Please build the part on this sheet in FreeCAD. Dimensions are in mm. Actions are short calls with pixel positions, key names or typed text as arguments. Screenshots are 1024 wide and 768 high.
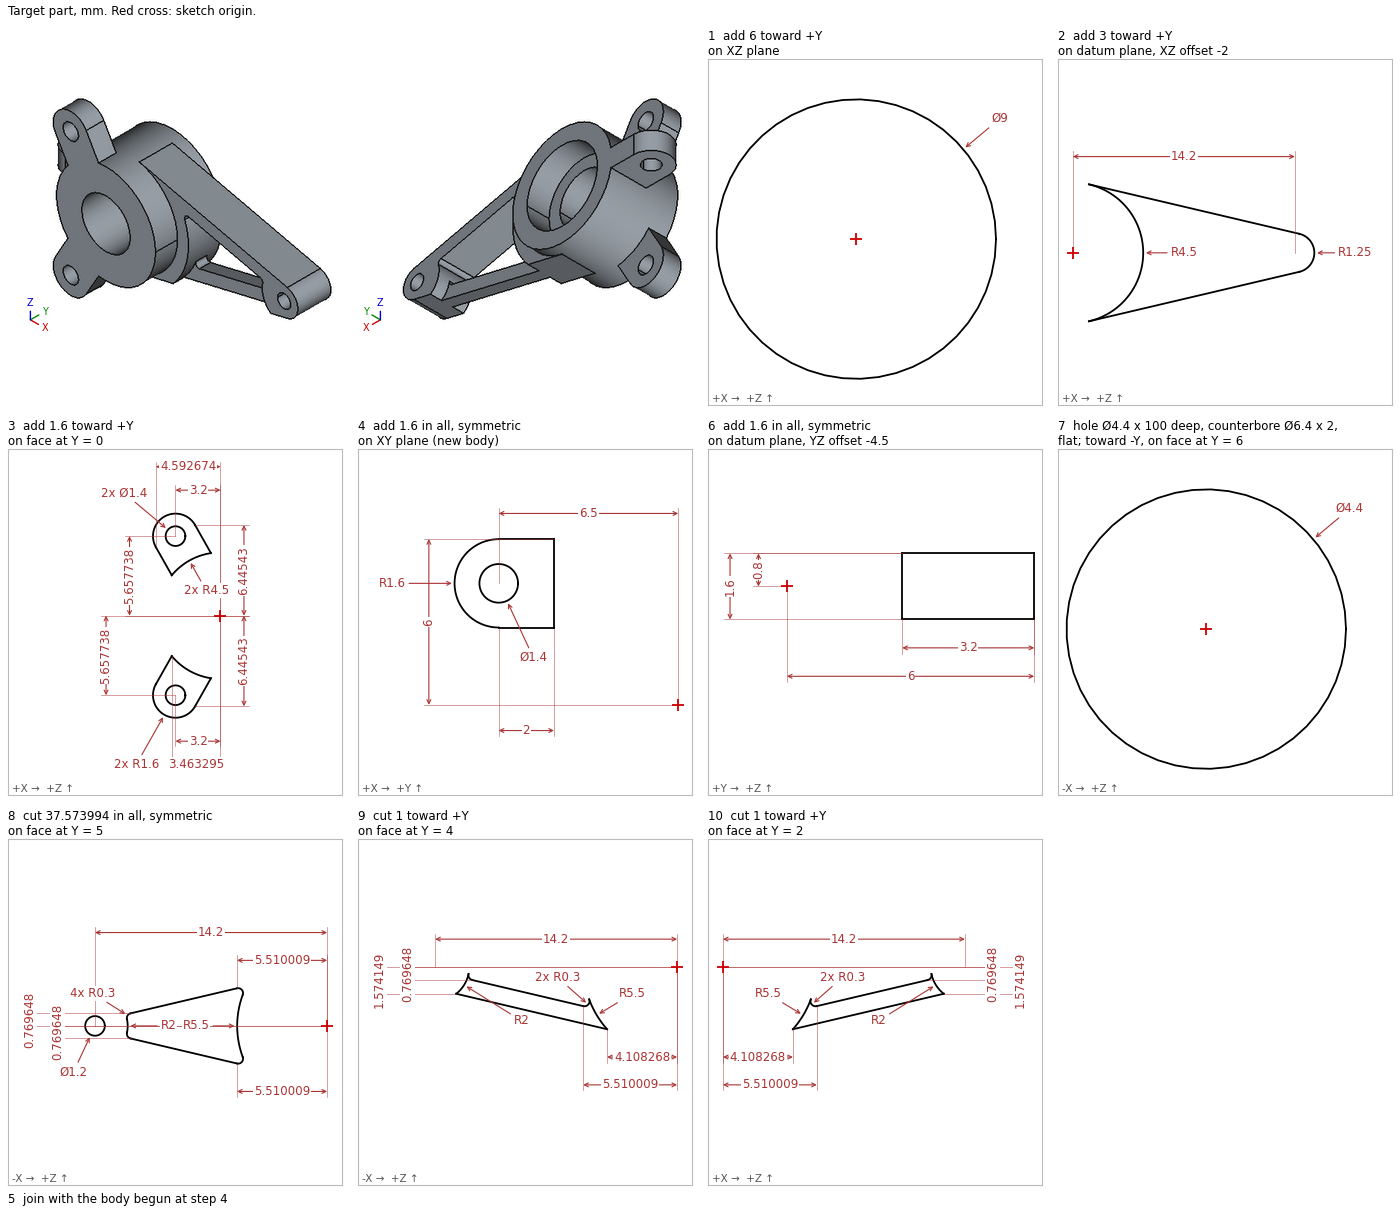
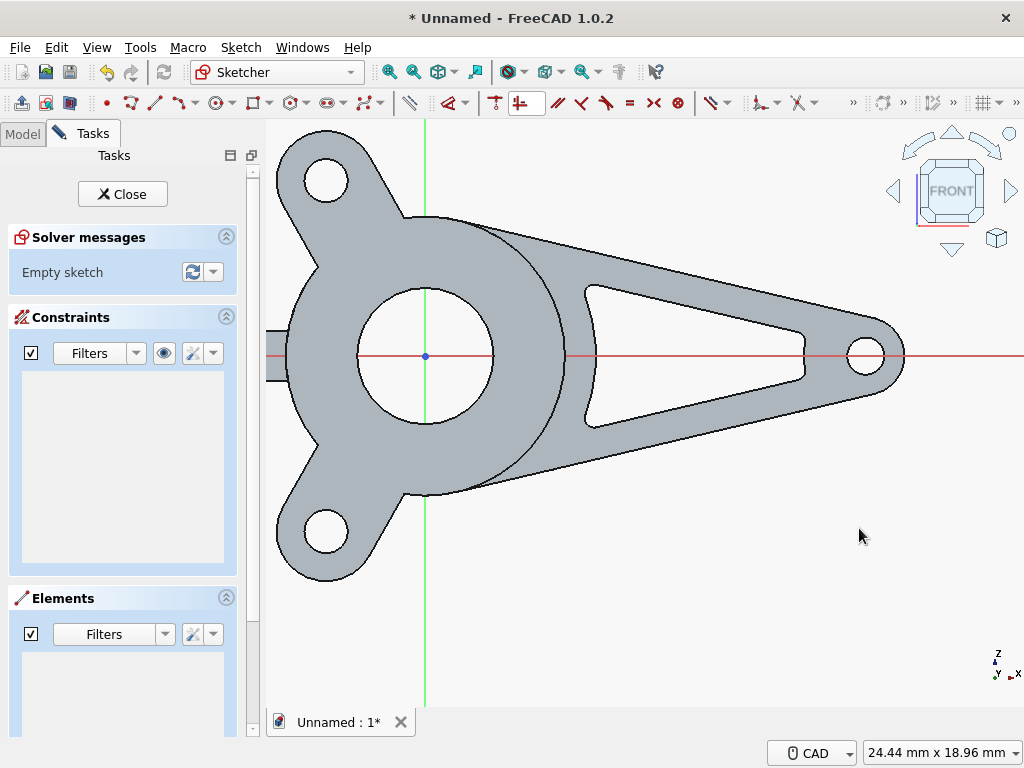
key(g)
key(l)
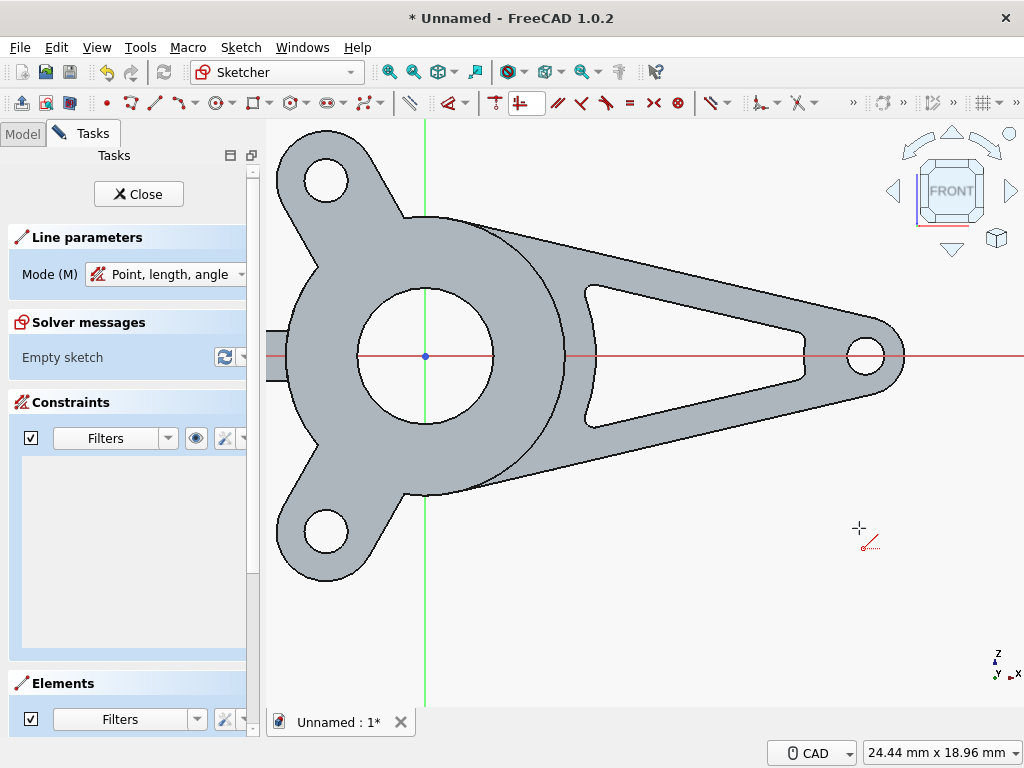
click(827, 405)
click(553, 470)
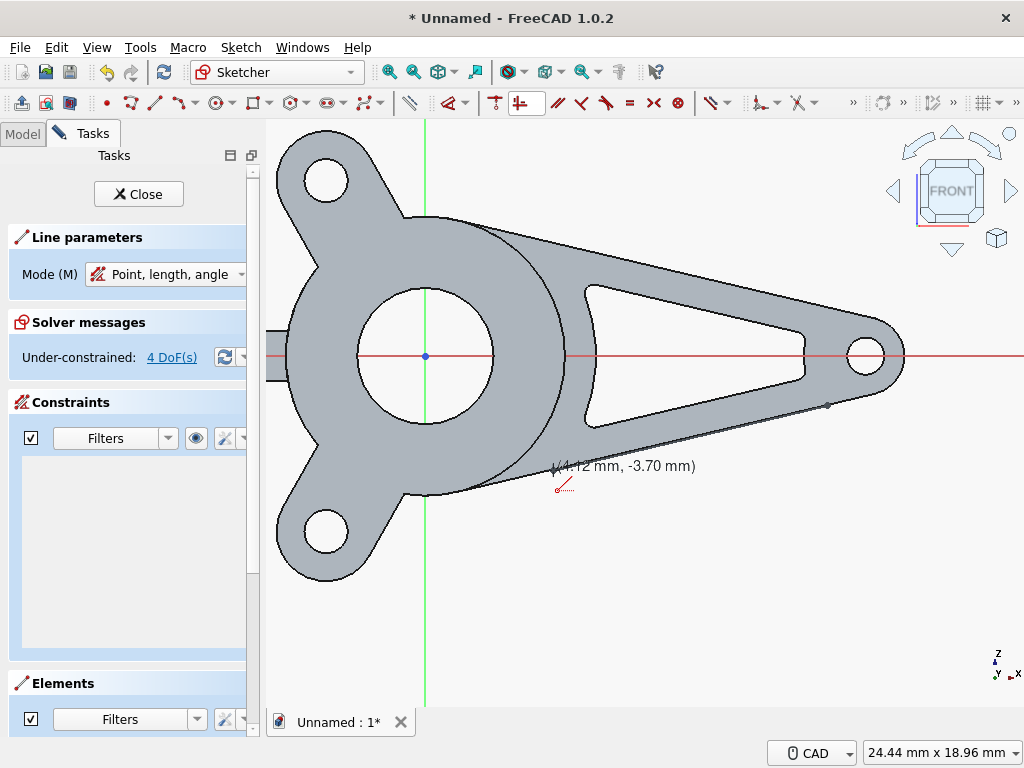
click(596, 427)
click(798, 380)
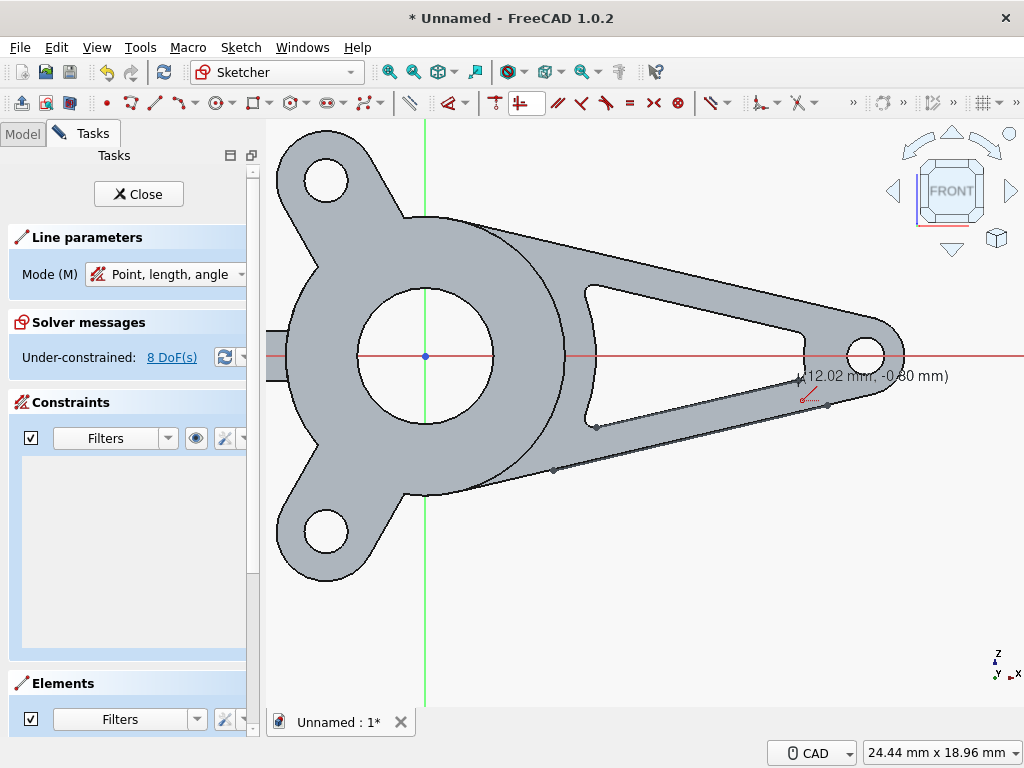
key(g)
key(3)
key(a)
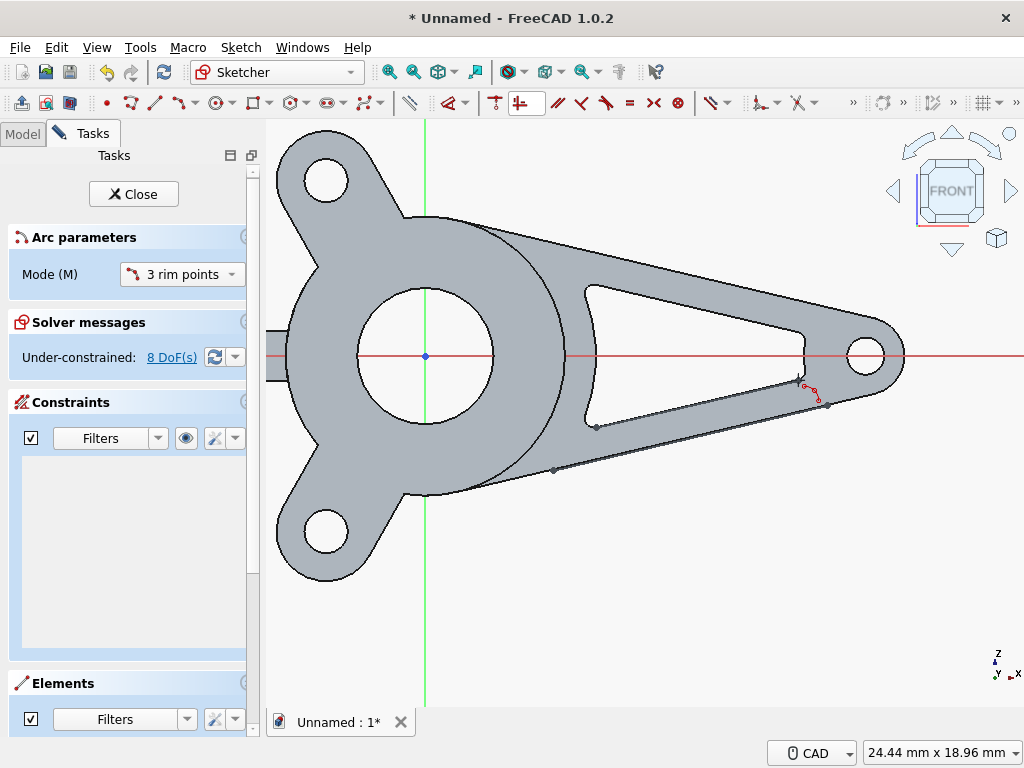
click(553, 471)
click(585, 415)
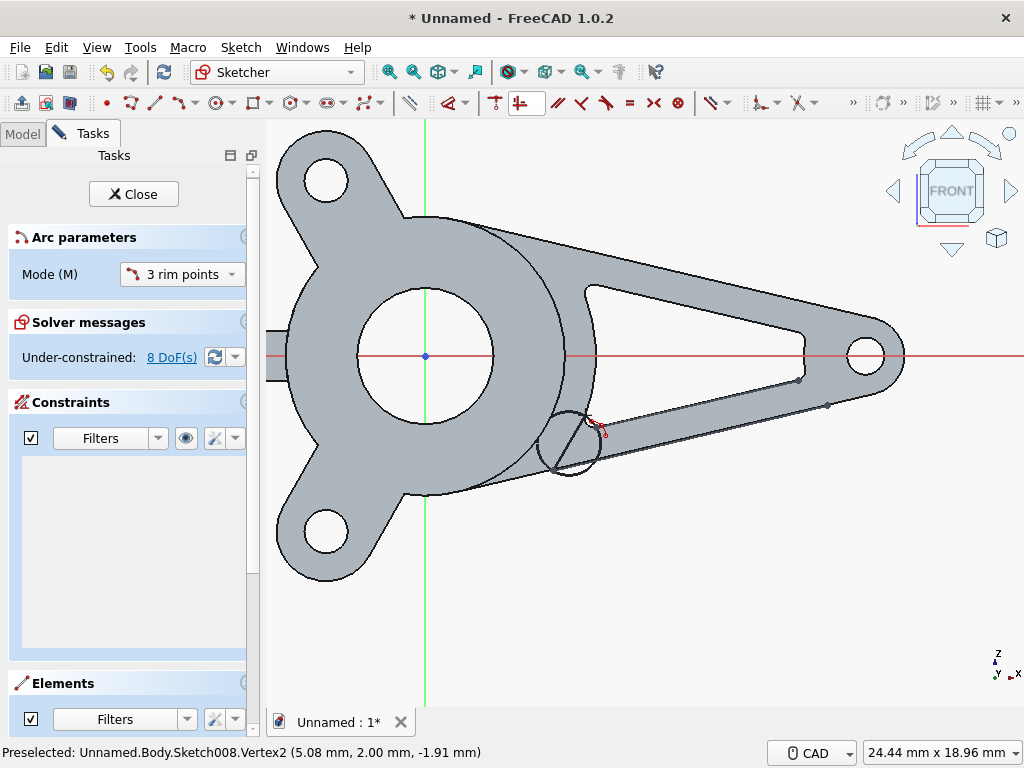
scroll(572, 444, up, 9)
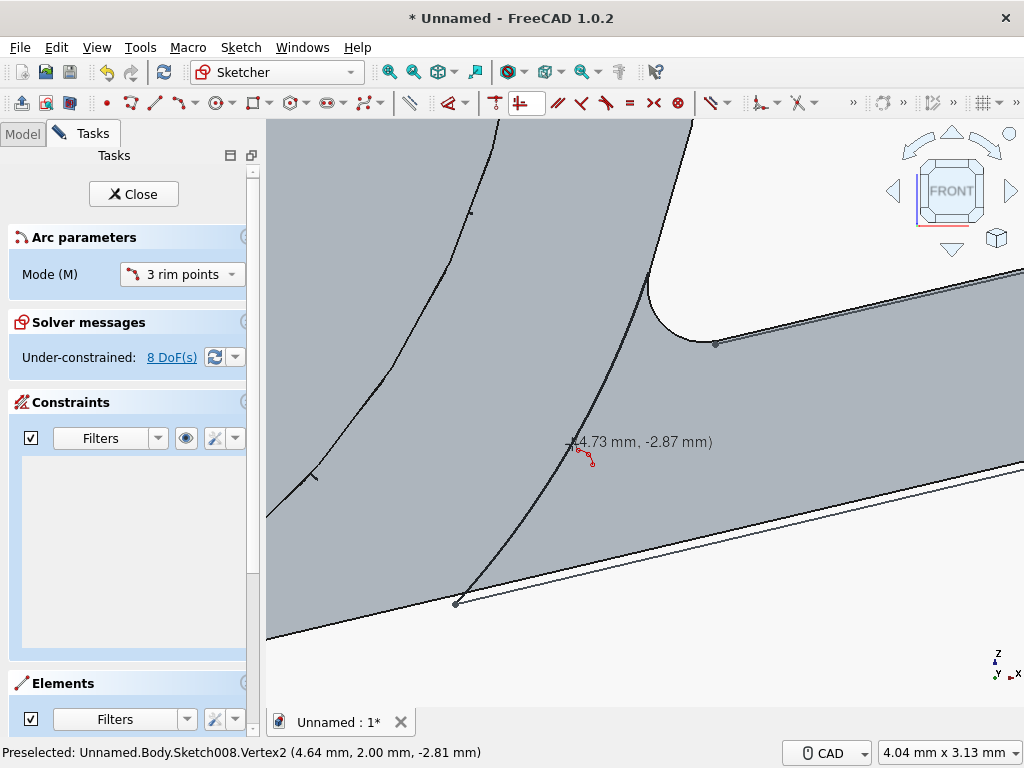
click(568, 440)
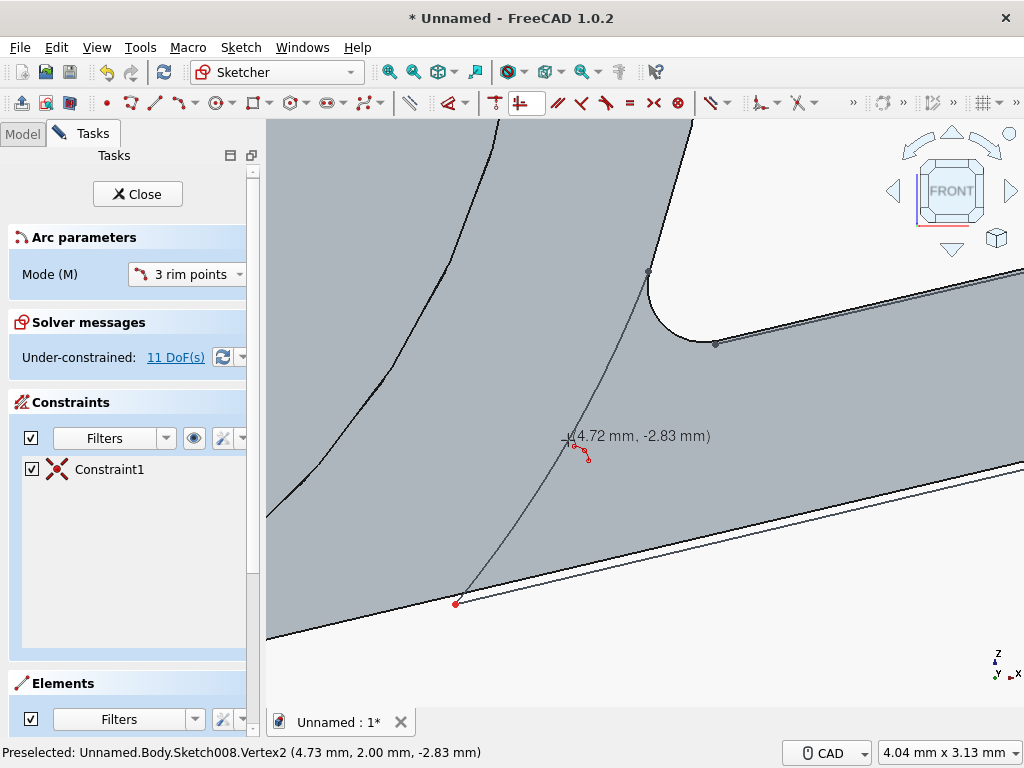
scroll(513, 445, down, 9)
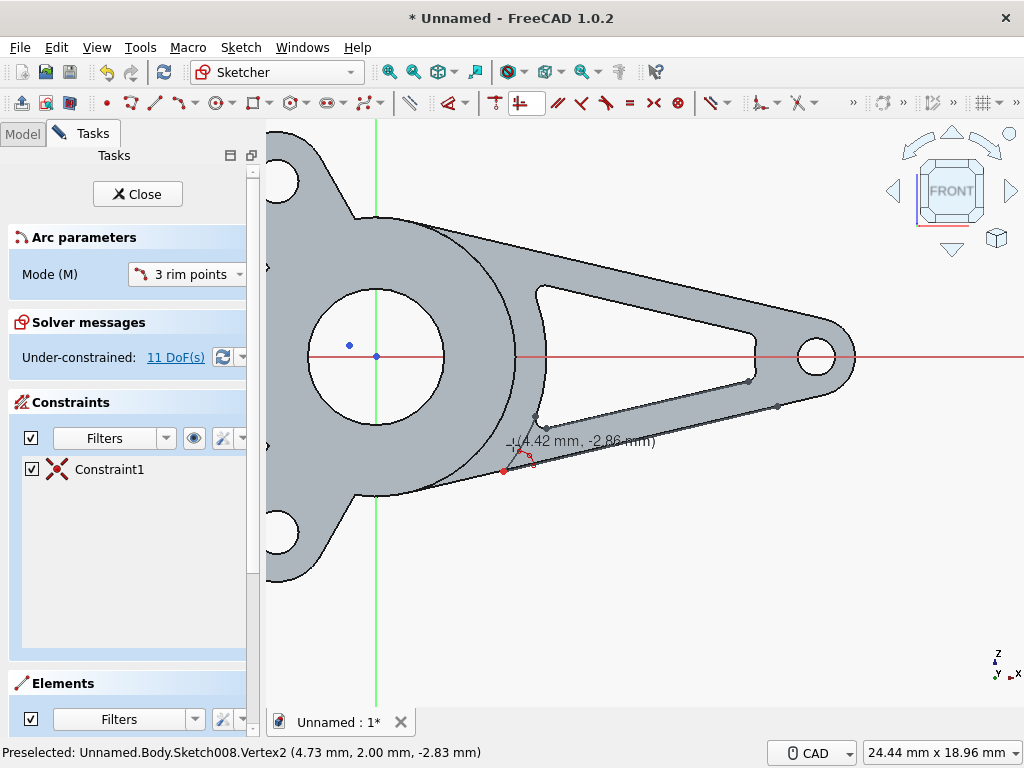
click(536, 417)
click(547, 429)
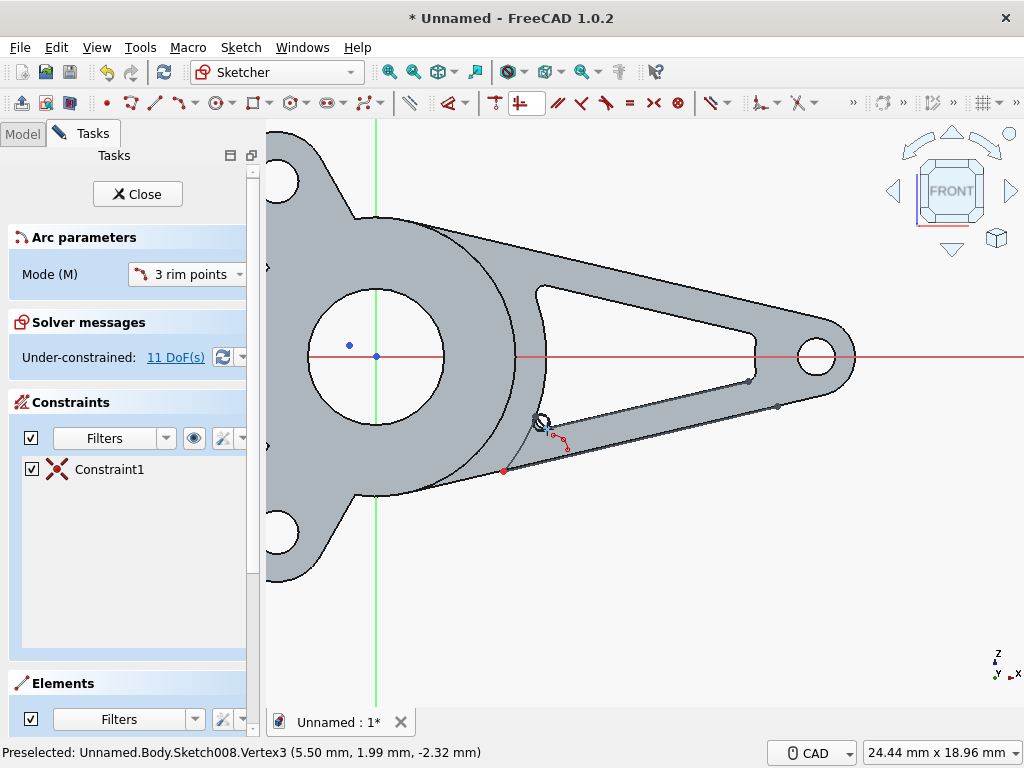
scroll(538, 425, up, 6)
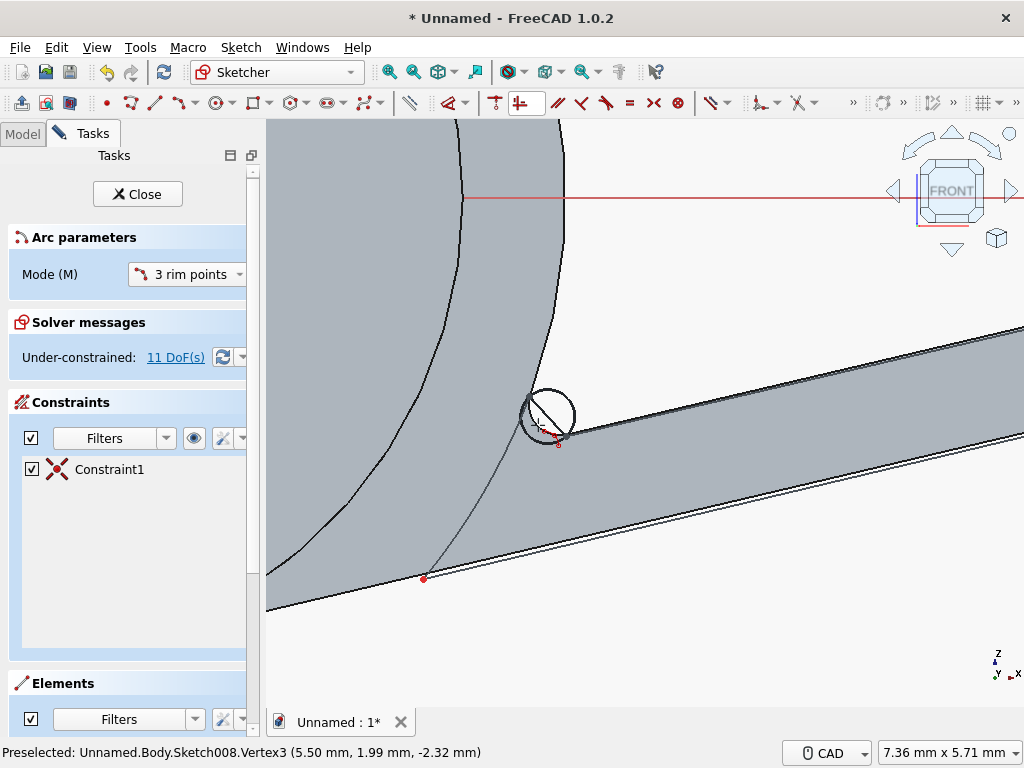
click(537, 425)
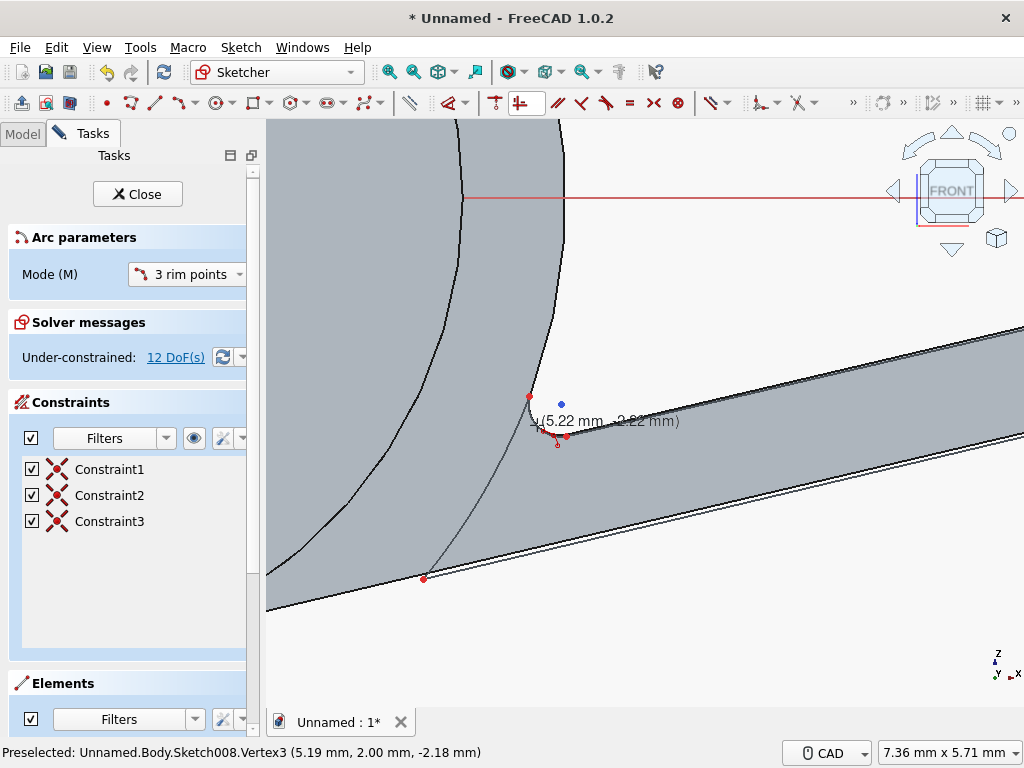
scroll(537, 425, down, 6)